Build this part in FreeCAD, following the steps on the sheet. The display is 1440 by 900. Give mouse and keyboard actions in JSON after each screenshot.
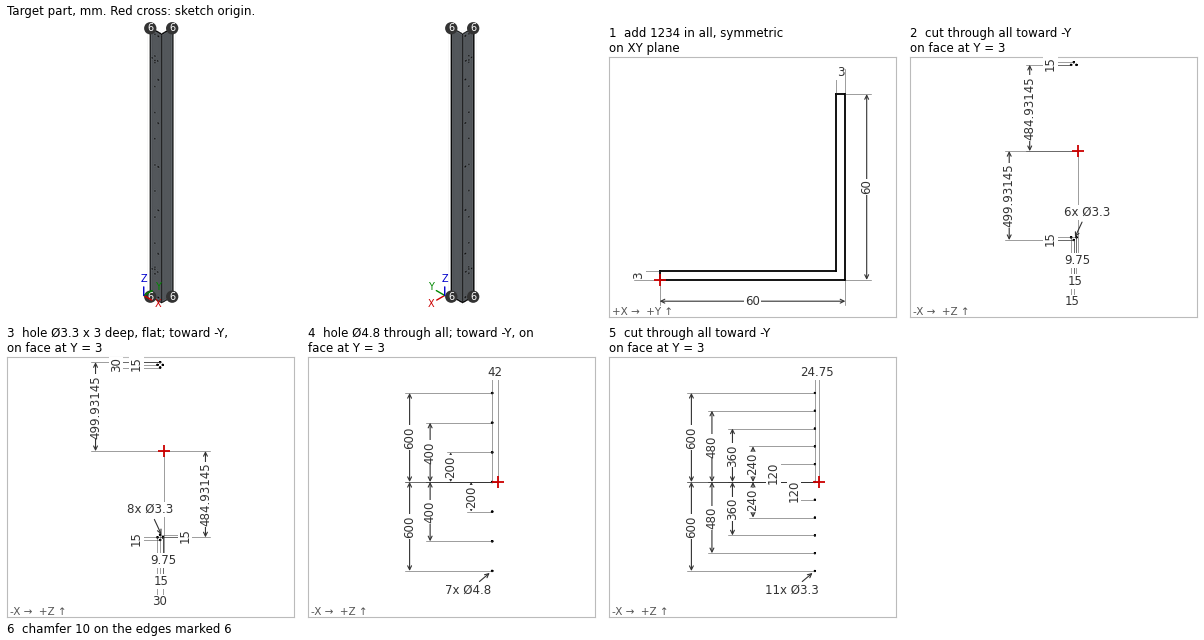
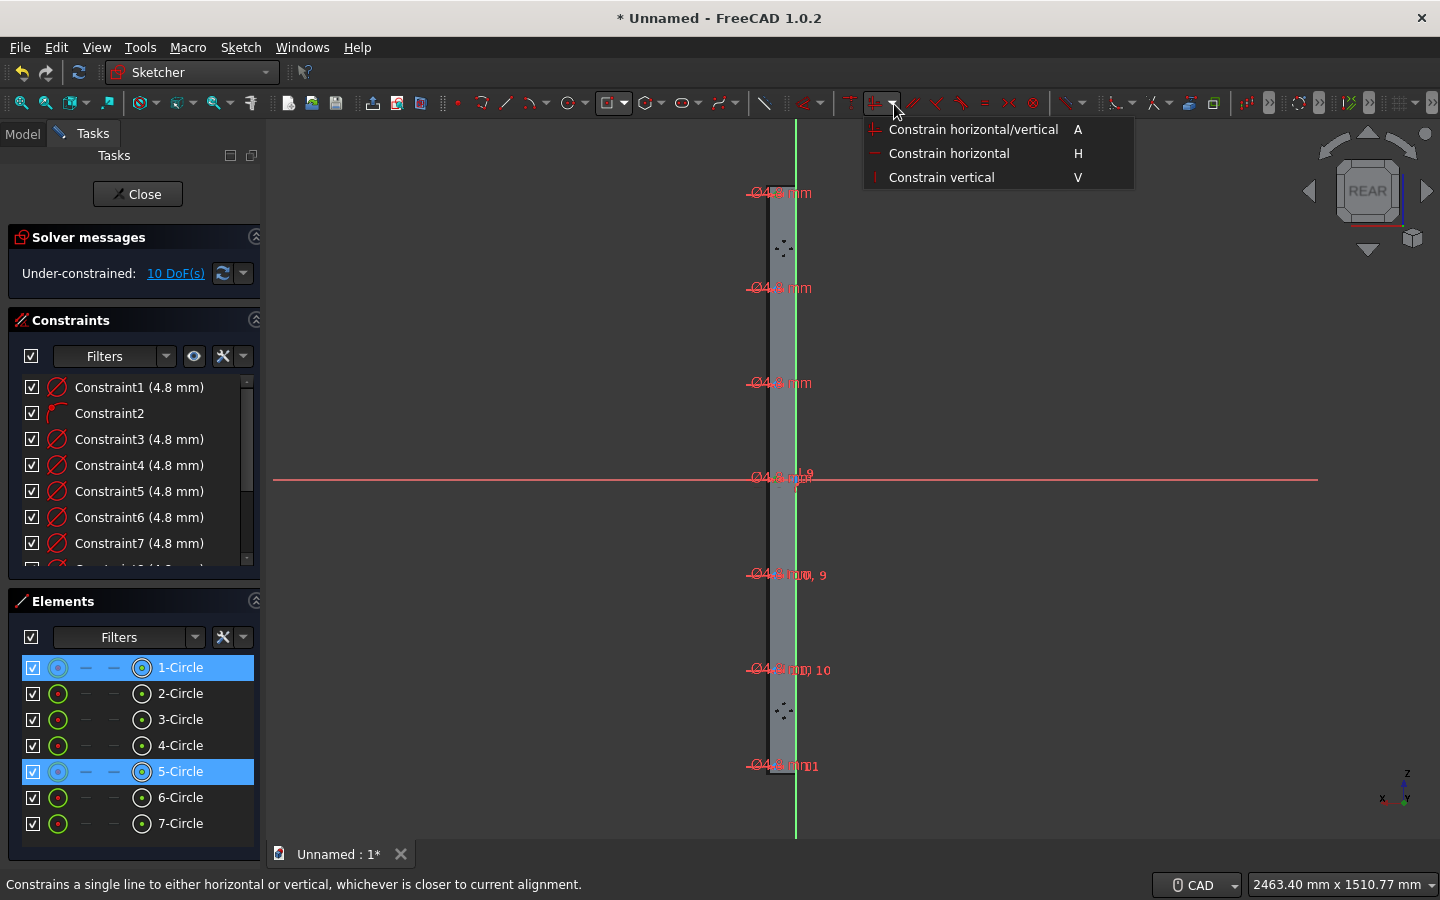
{"action": "left_click", "coordinate": [999, 177]}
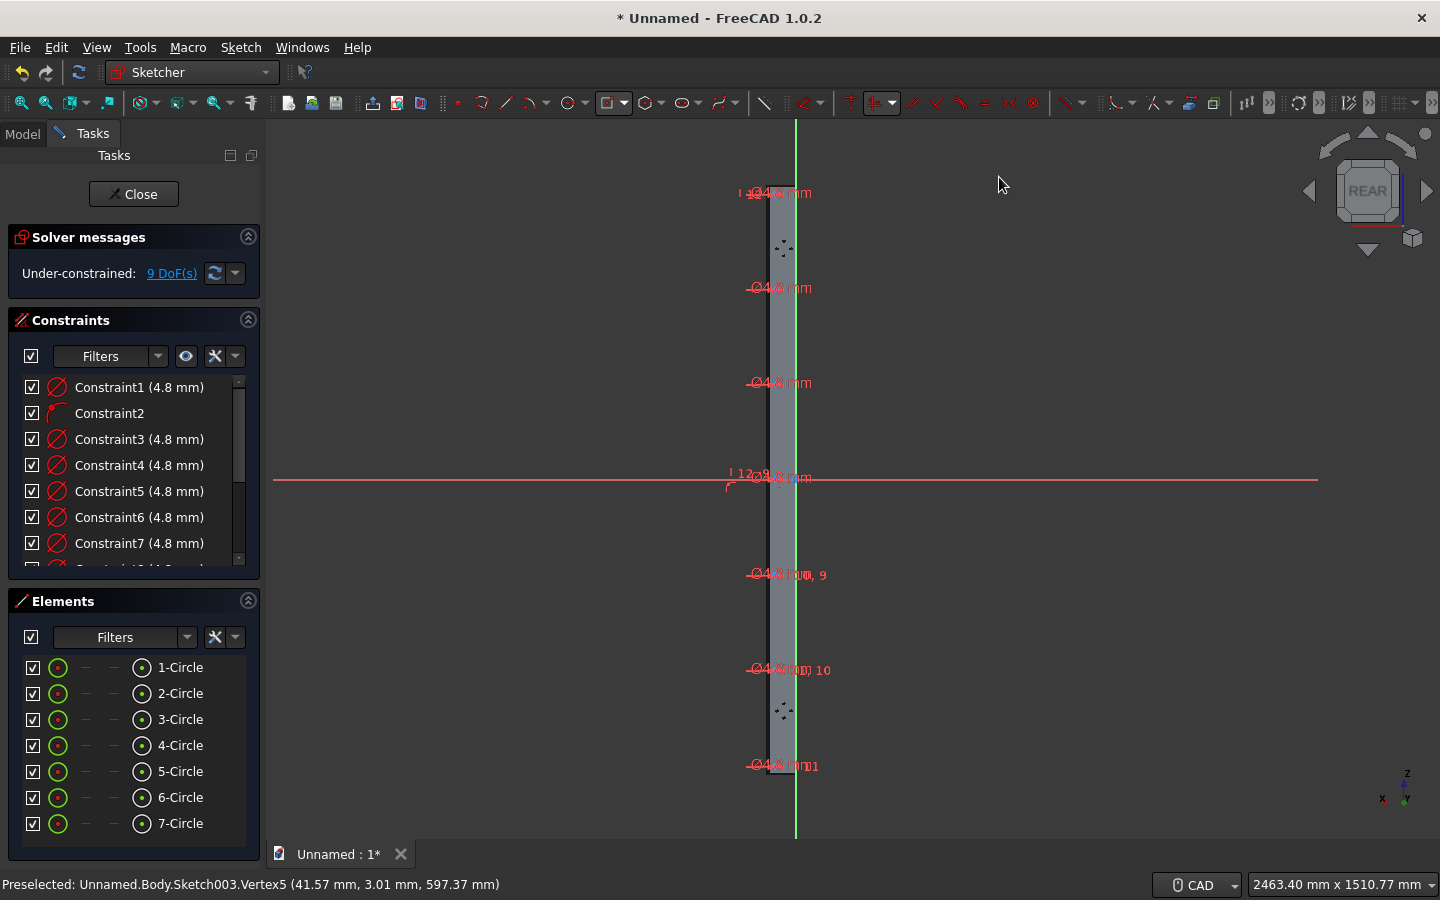
{"action": "left_click", "coordinate": [776, 195]}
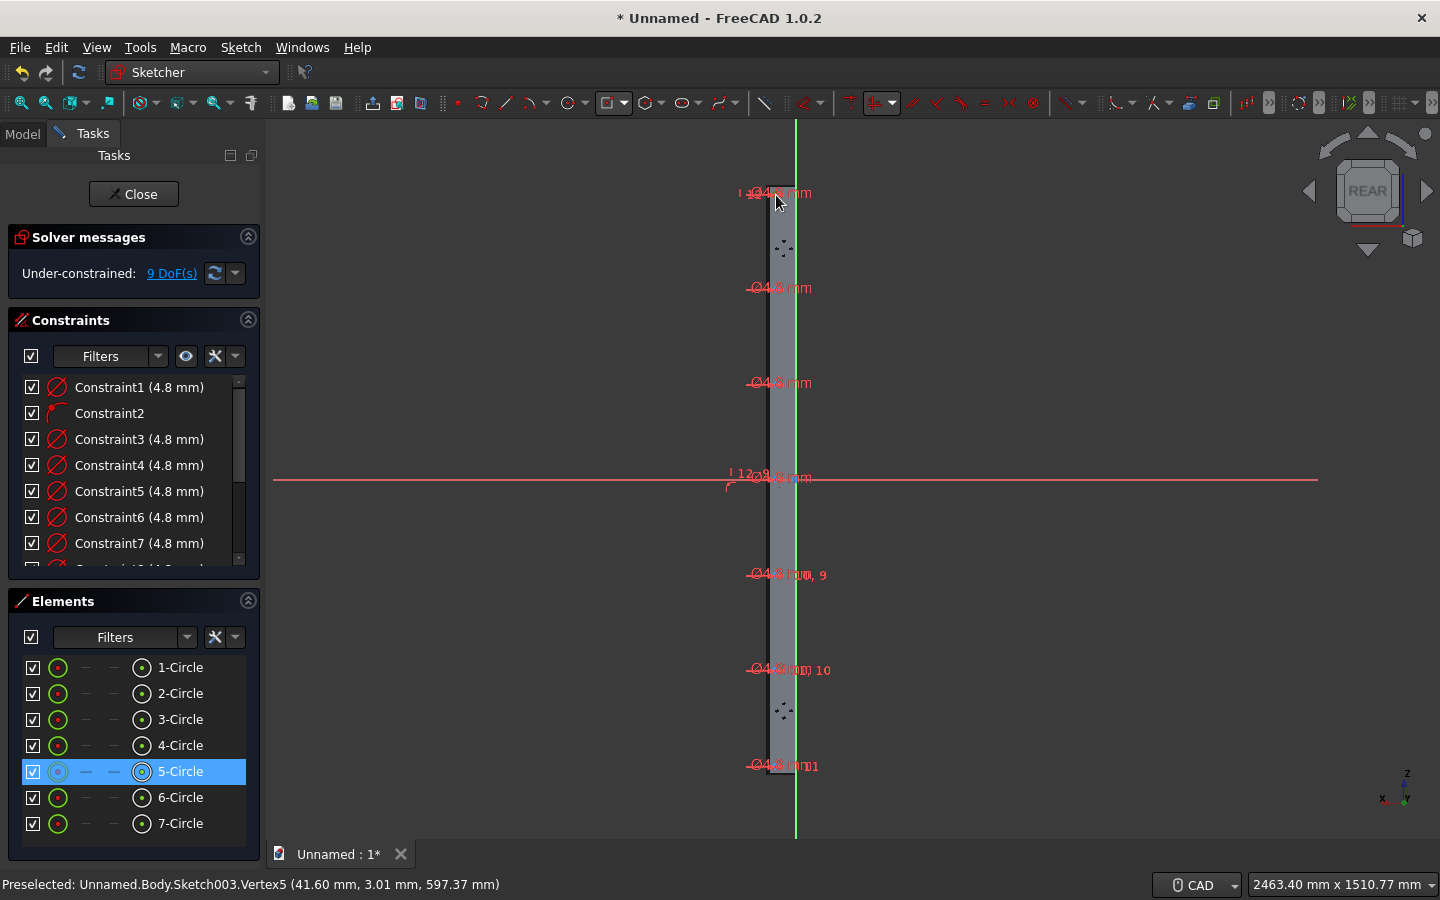
{"action": "left_click", "coordinate": [776, 290]}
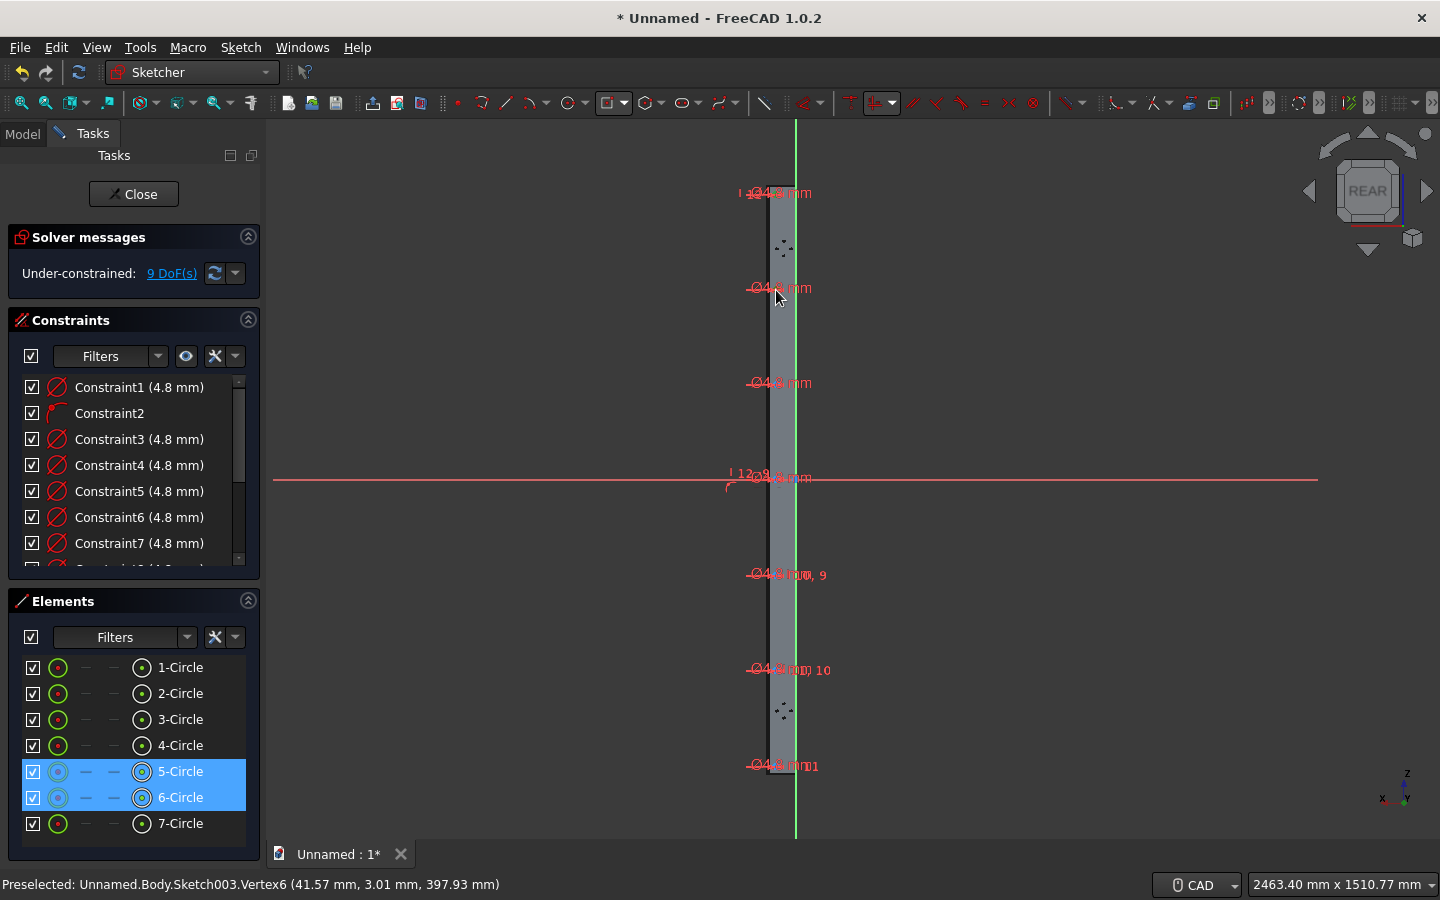
{"action": "key", "text": "v"}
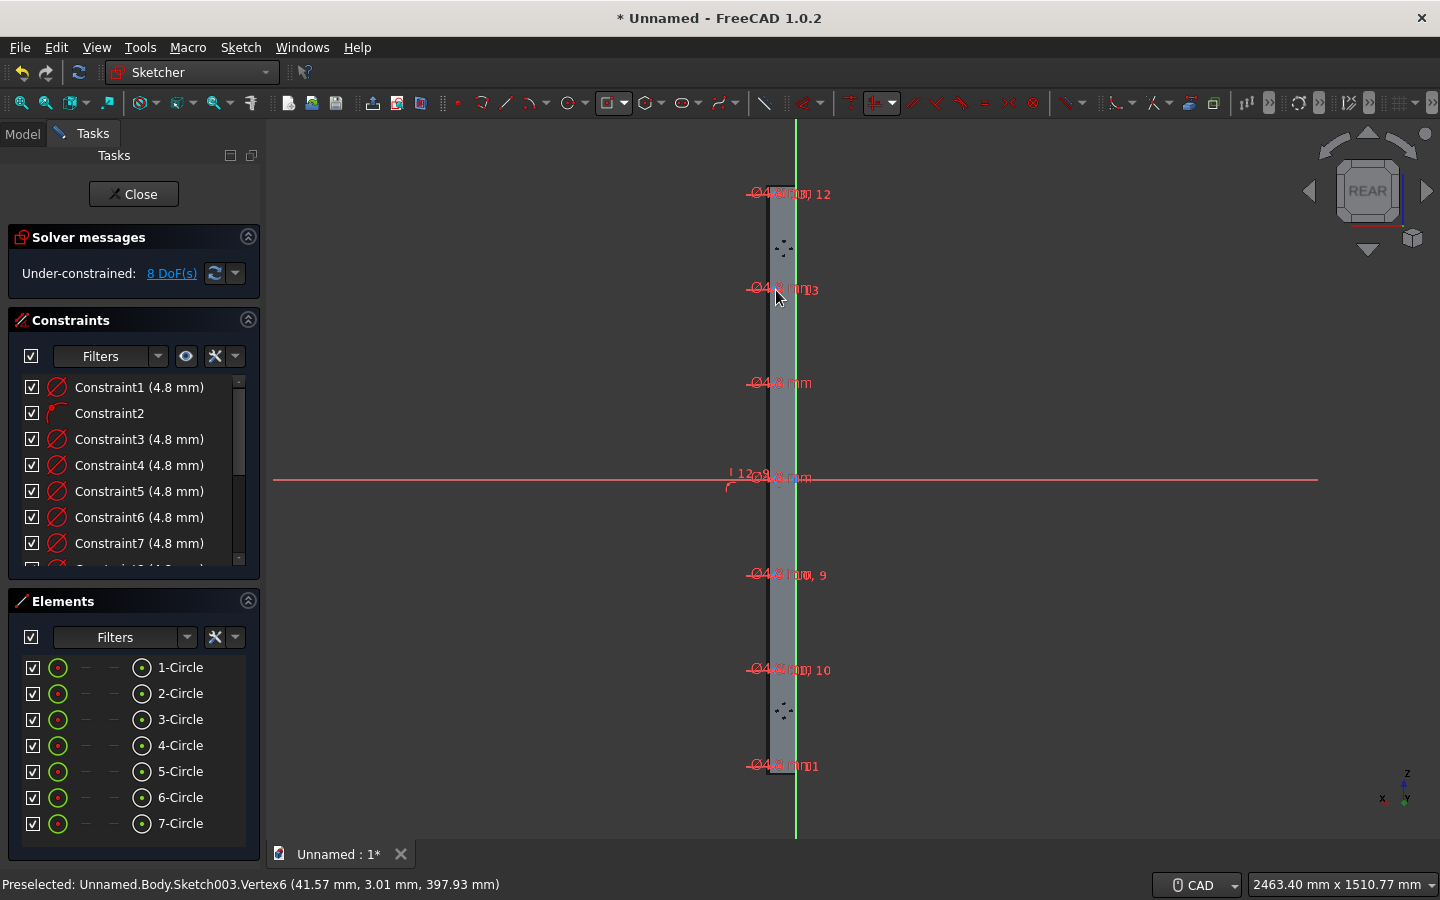
{"action": "left_click", "coordinate": [776, 480]}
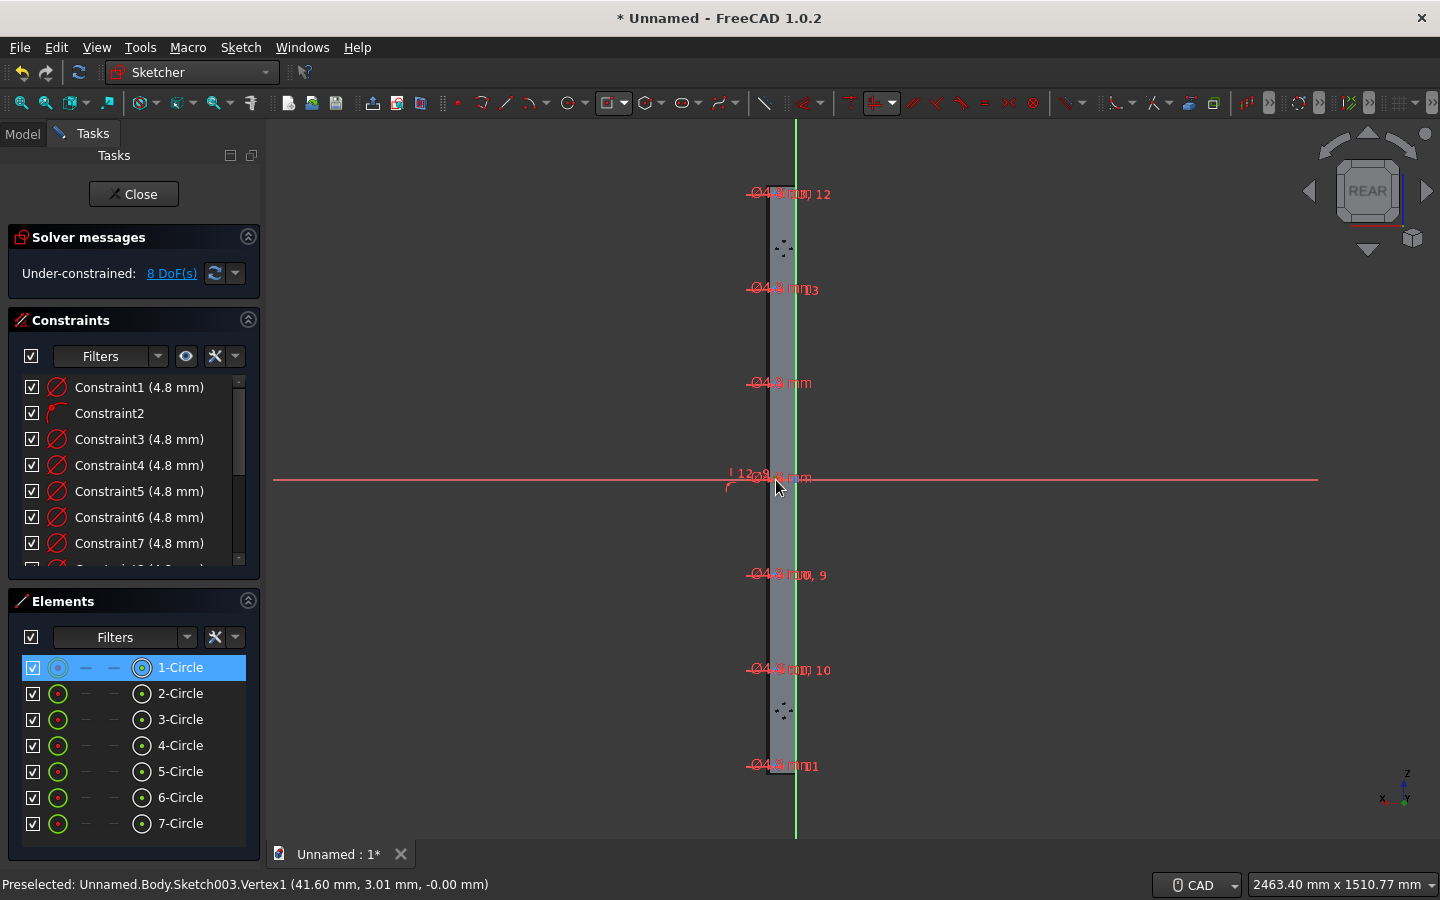
{"action": "left_click", "coordinate": [776, 385]}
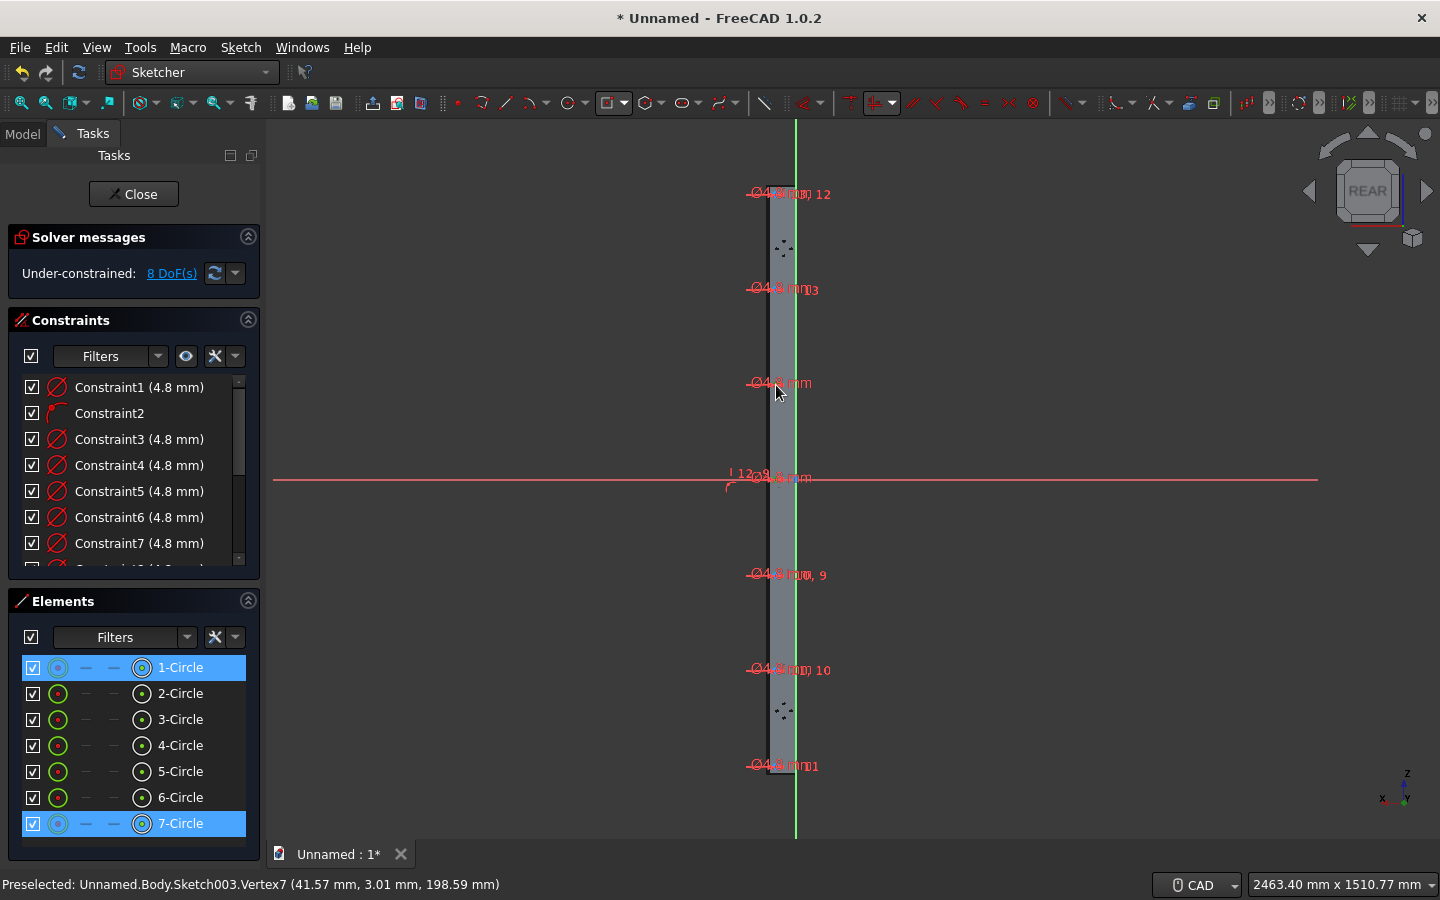
{"action": "key", "text": "v"}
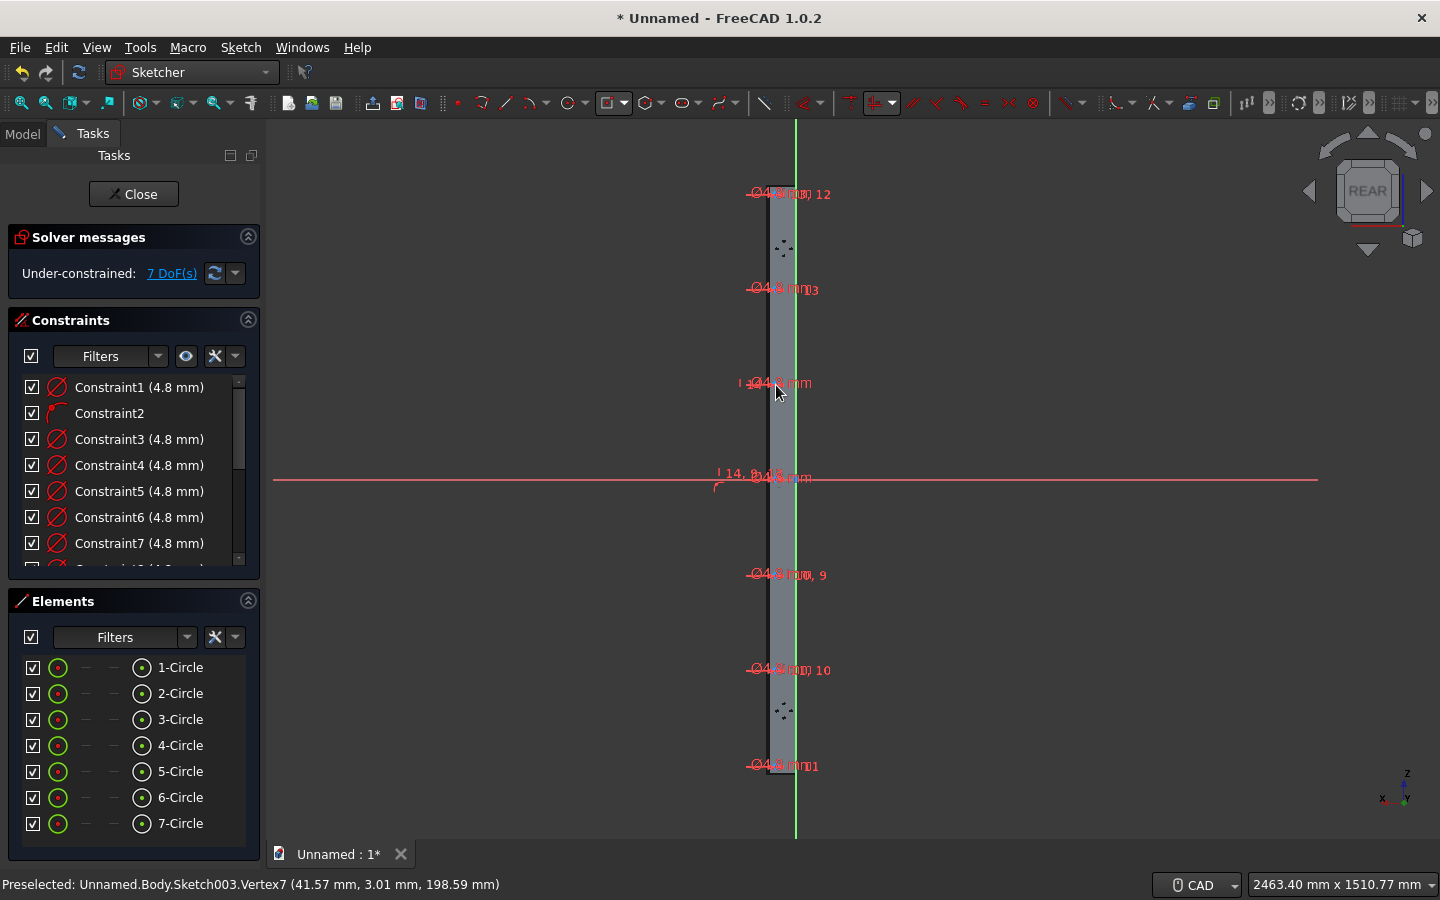
{"action": "left_click", "coordinate": [804, 104]}